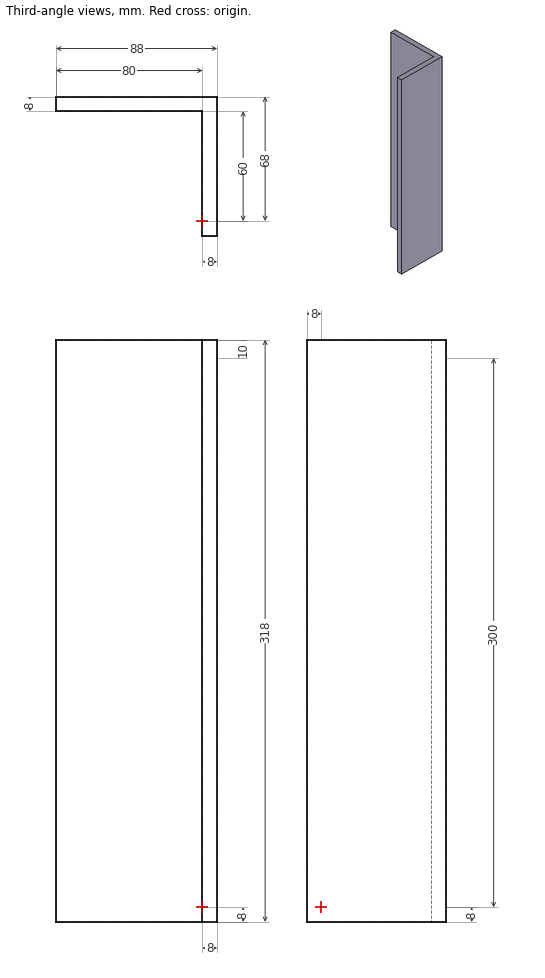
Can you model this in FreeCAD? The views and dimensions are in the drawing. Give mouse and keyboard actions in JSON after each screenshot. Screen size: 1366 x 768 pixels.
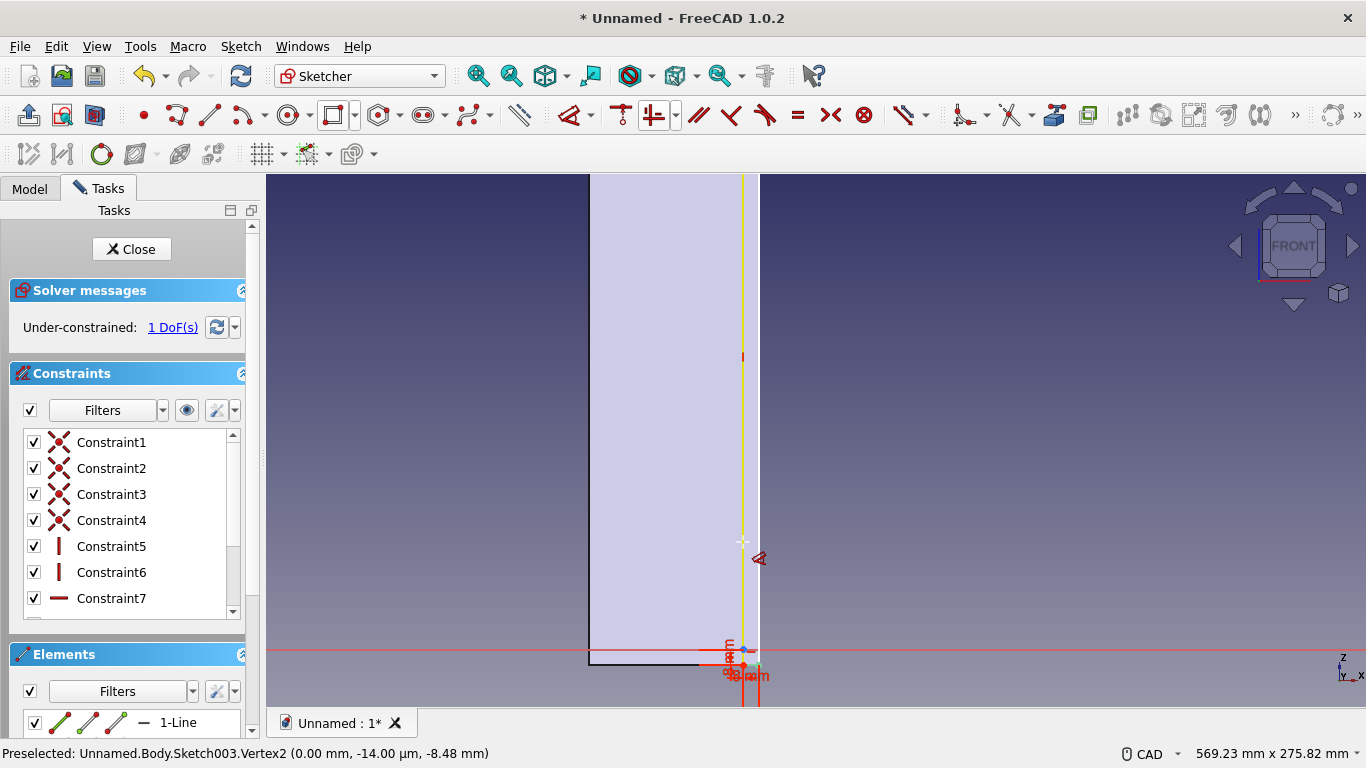
{"action": "left_click", "coordinate": [743, 542]}
{"action": "left_click", "coordinate": [709, 434]}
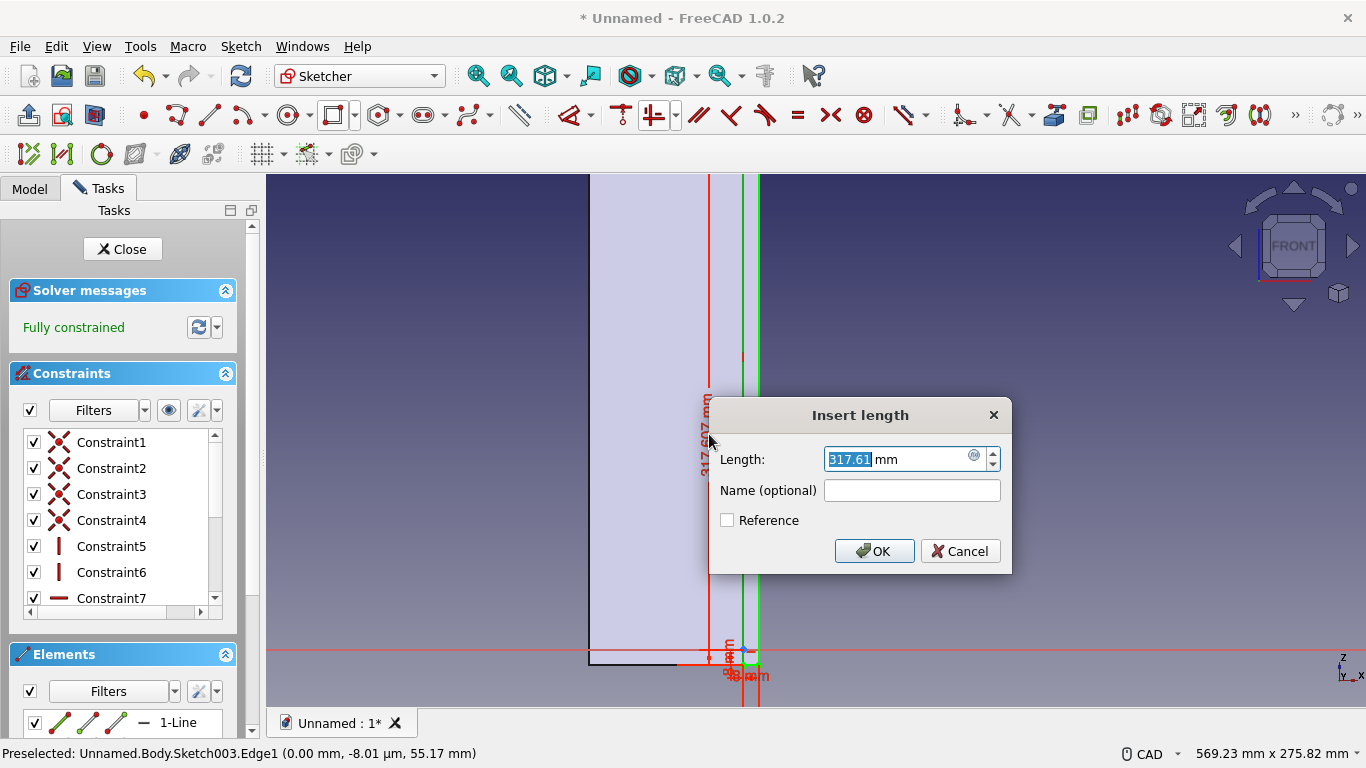
{"action": "type", "text": "318"}
{"action": "key", "text": "Return"}
{"action": "key", "text": "Escape"}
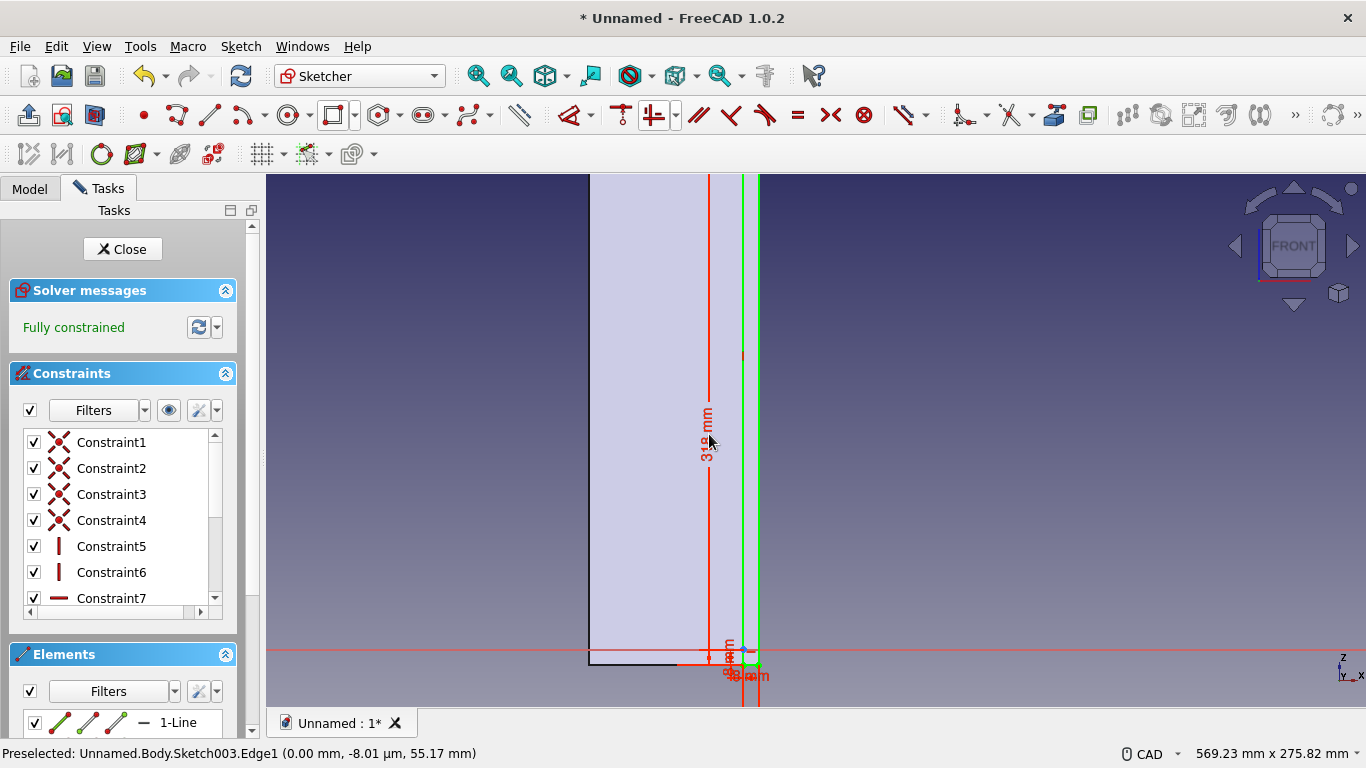
{"action": "left_click", "coordinate": [123, 249]}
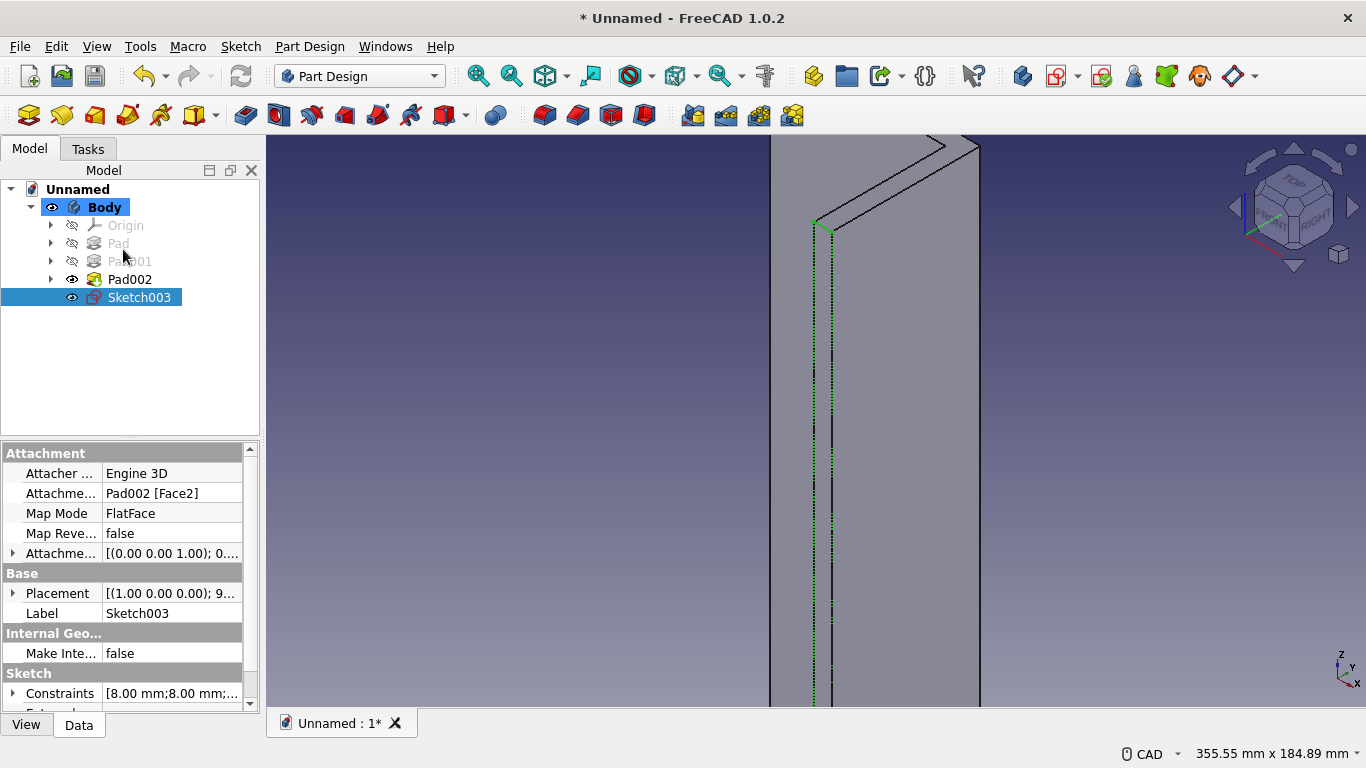
{"action": "left_click", "coordinate": [29, 116]}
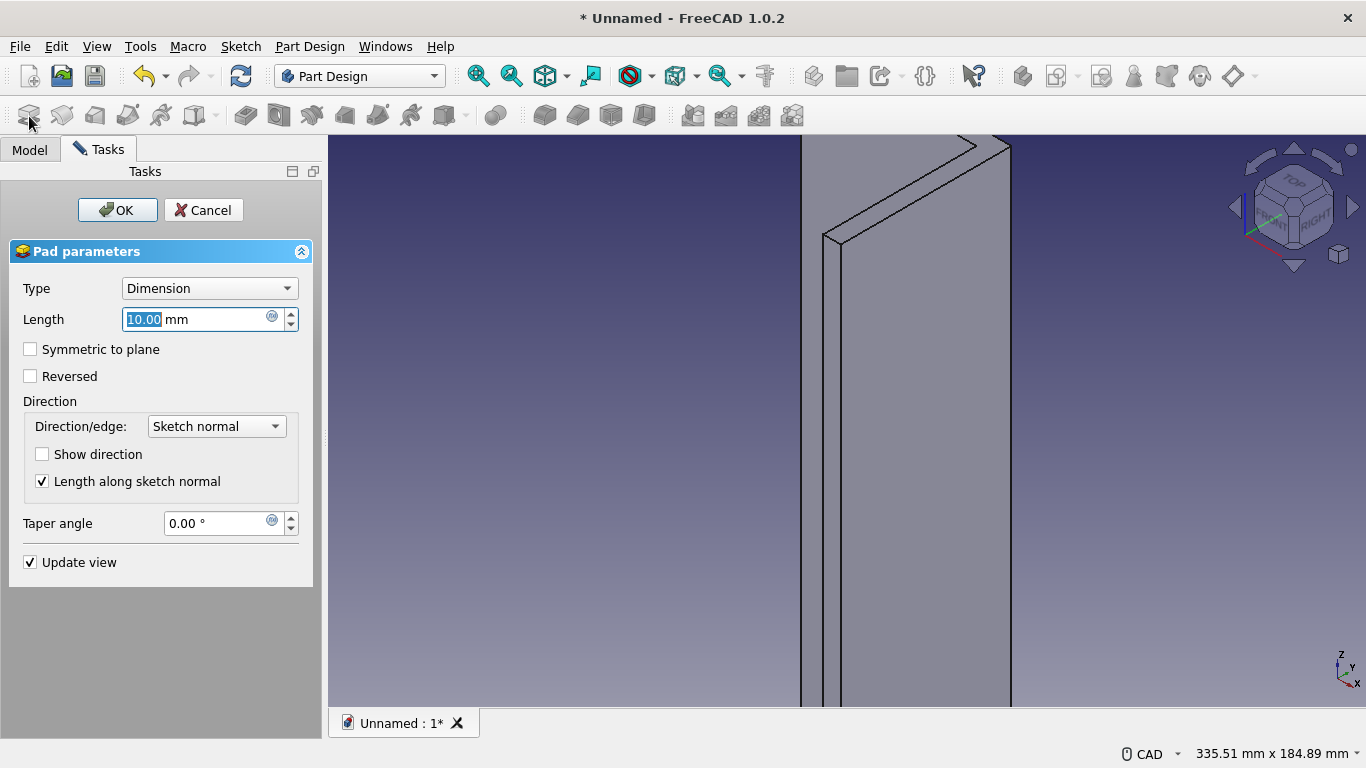
{"action": "type", "text": "8"}
{"action": "key", "text": "Tab"}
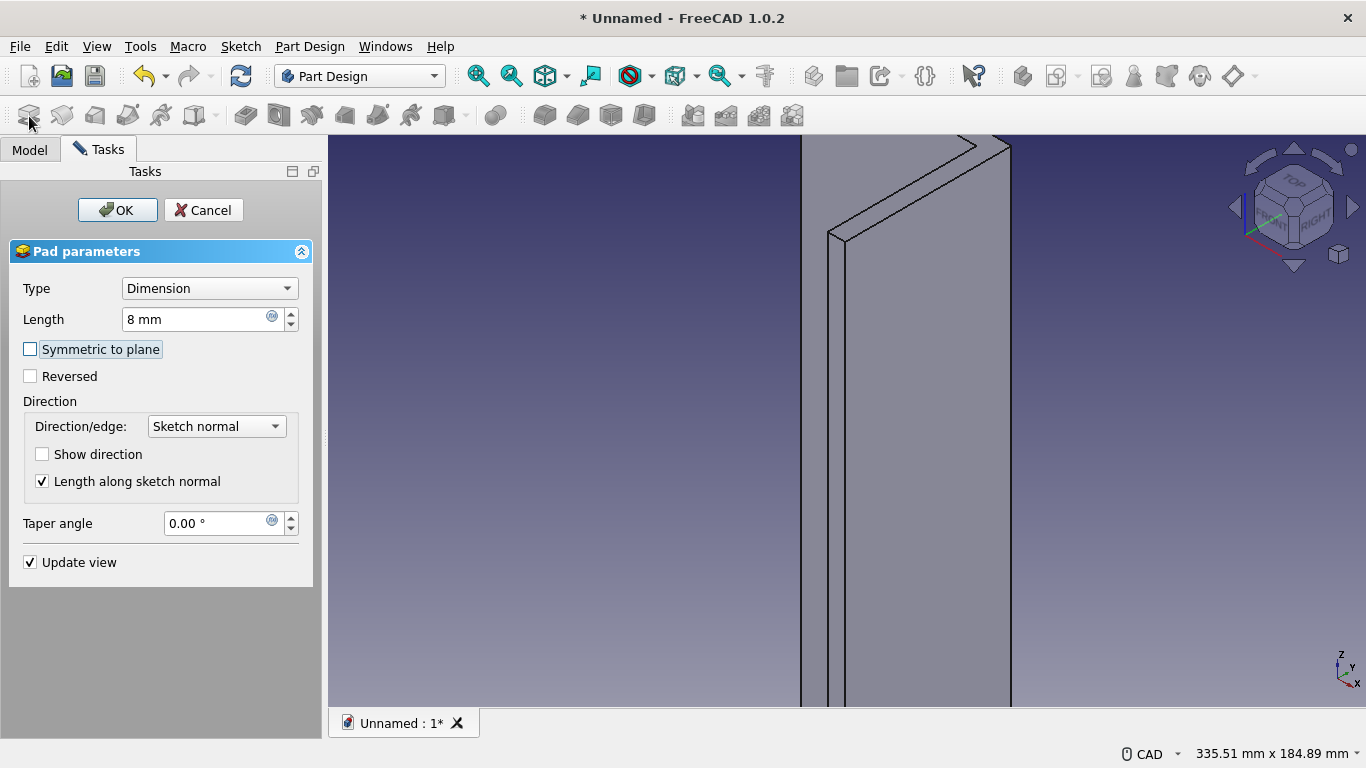
{"action": "left_click", "coordinate": [118, 210]}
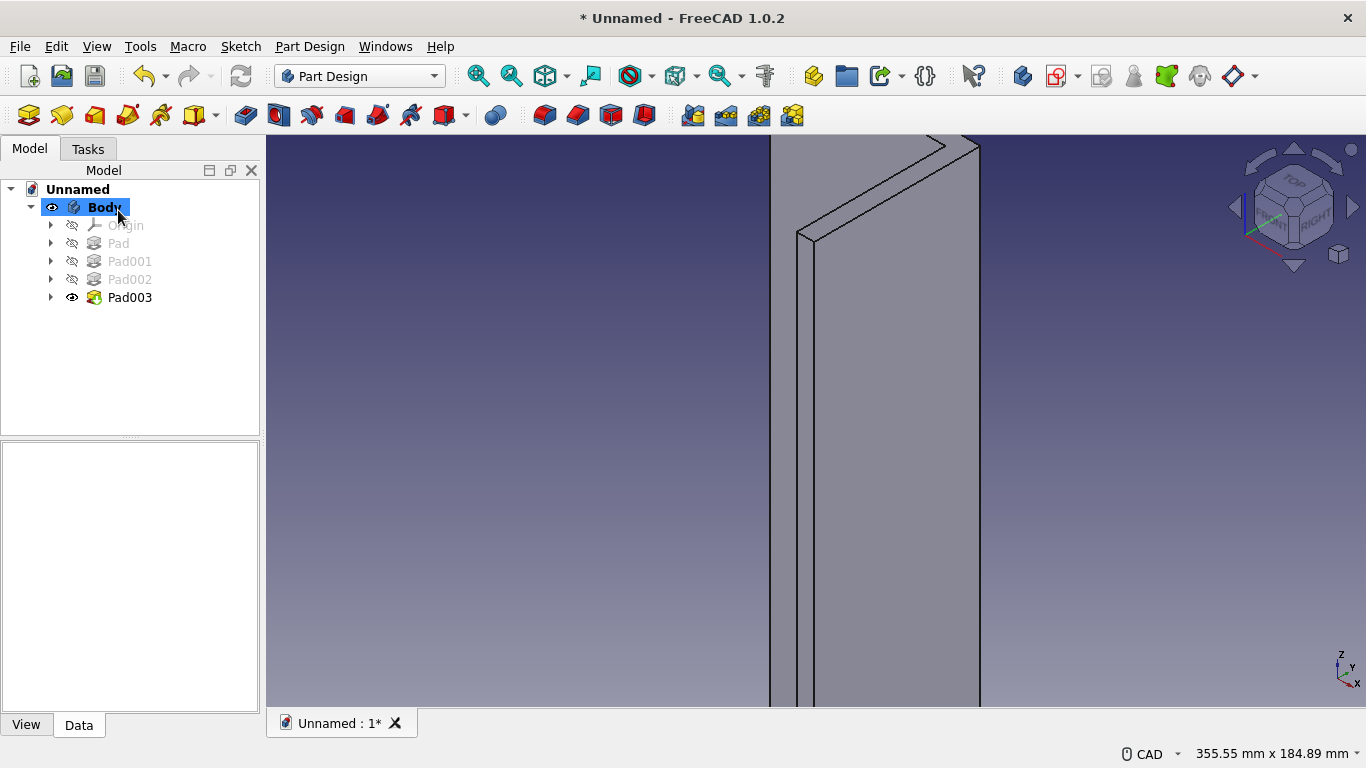
{"action": "key", "text": "v f"}